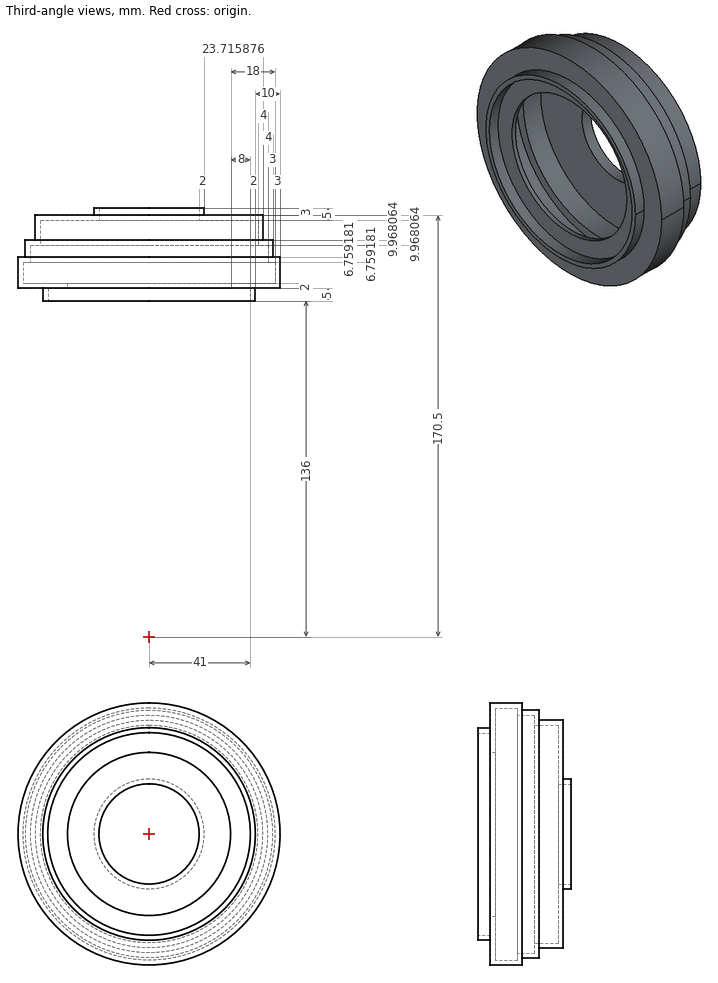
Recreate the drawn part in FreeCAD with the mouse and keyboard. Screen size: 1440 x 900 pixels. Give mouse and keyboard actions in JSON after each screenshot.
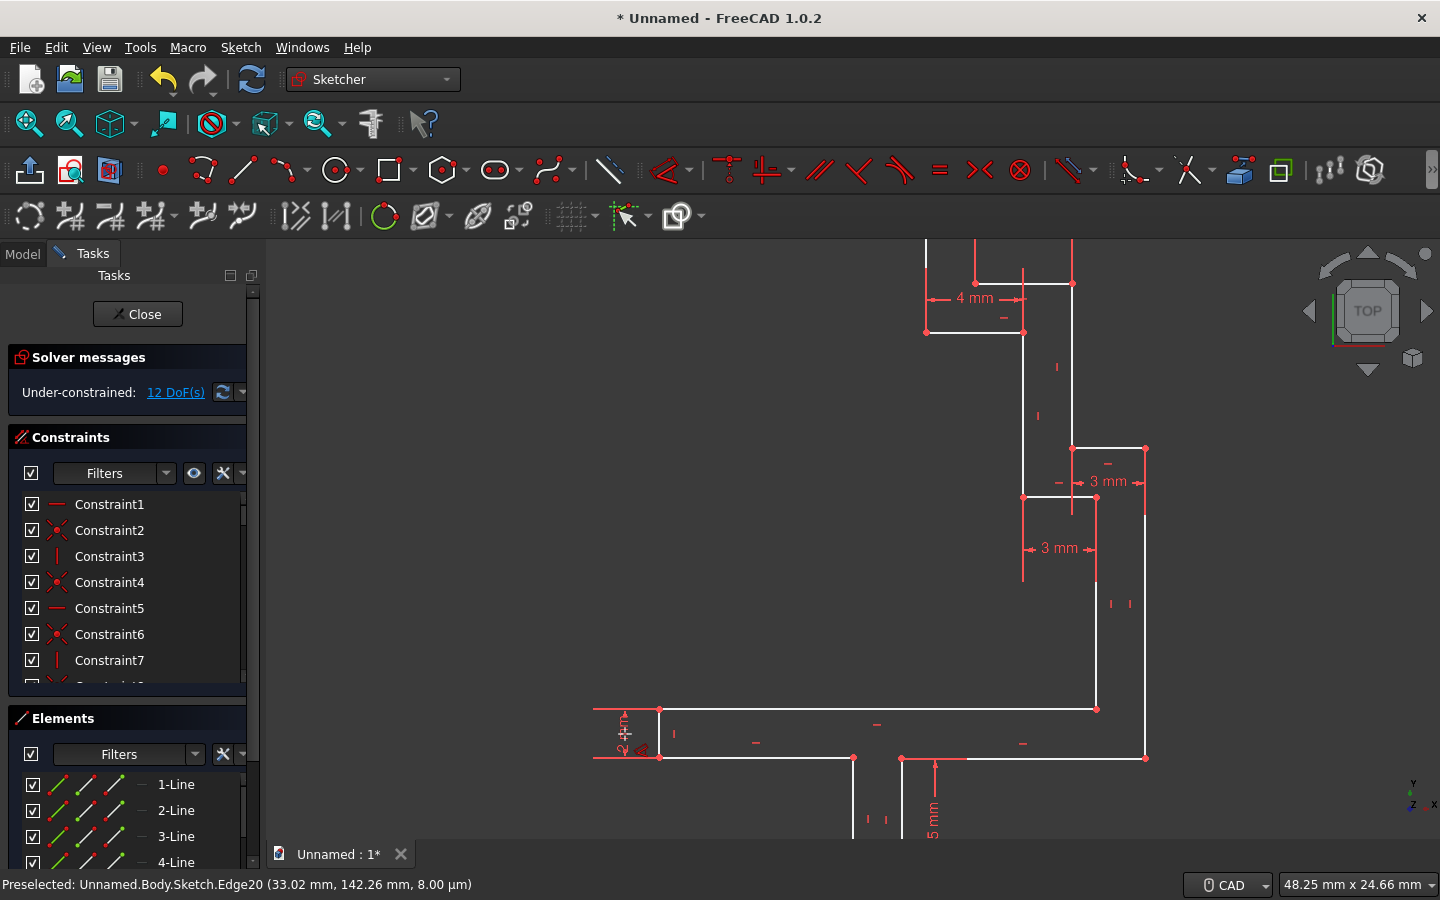
{"action": "left_click", "coordinate": [717, 758]}
{"action": "left_click", "coordinate": [756, 792]}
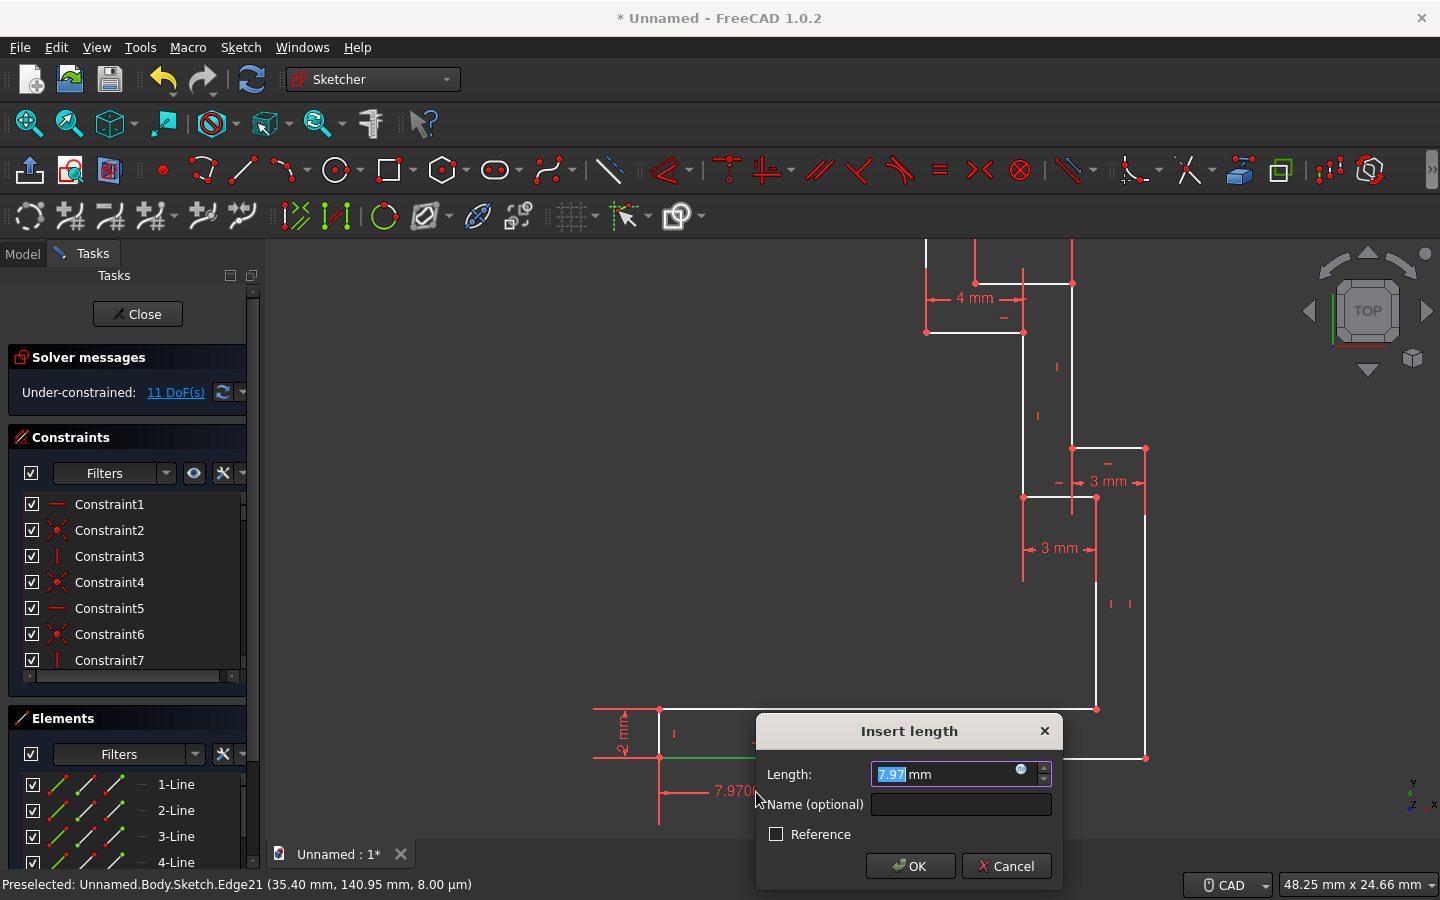
{"action": "type", "text": "8"}
{"action": "key", "text": "Return"}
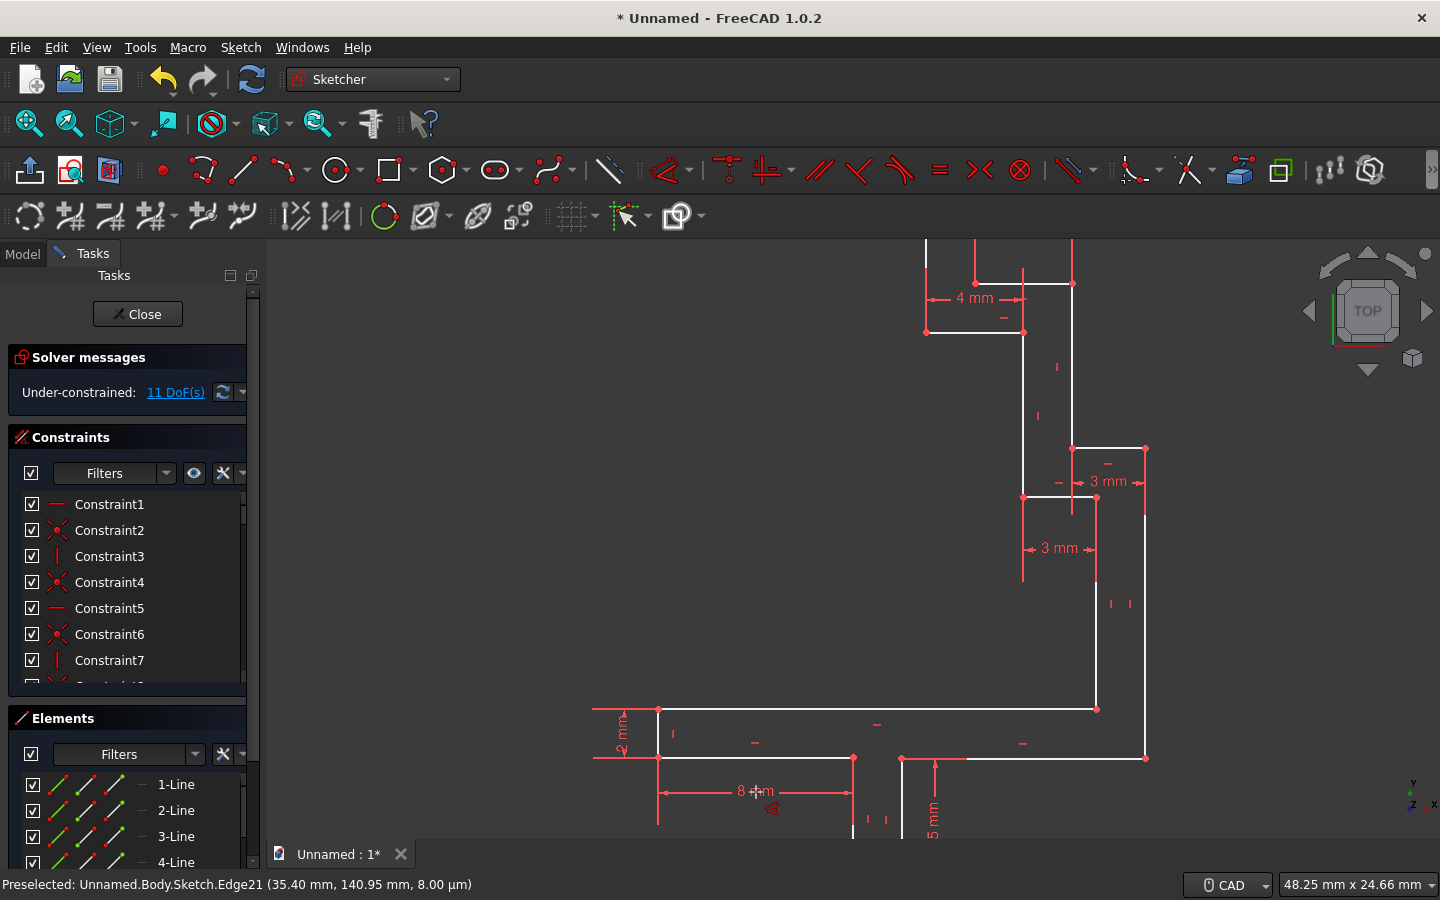
{"action": "left_click", "coordinate": [853, 794]}
{"action": "left_click", "coordinate": [887, 784]}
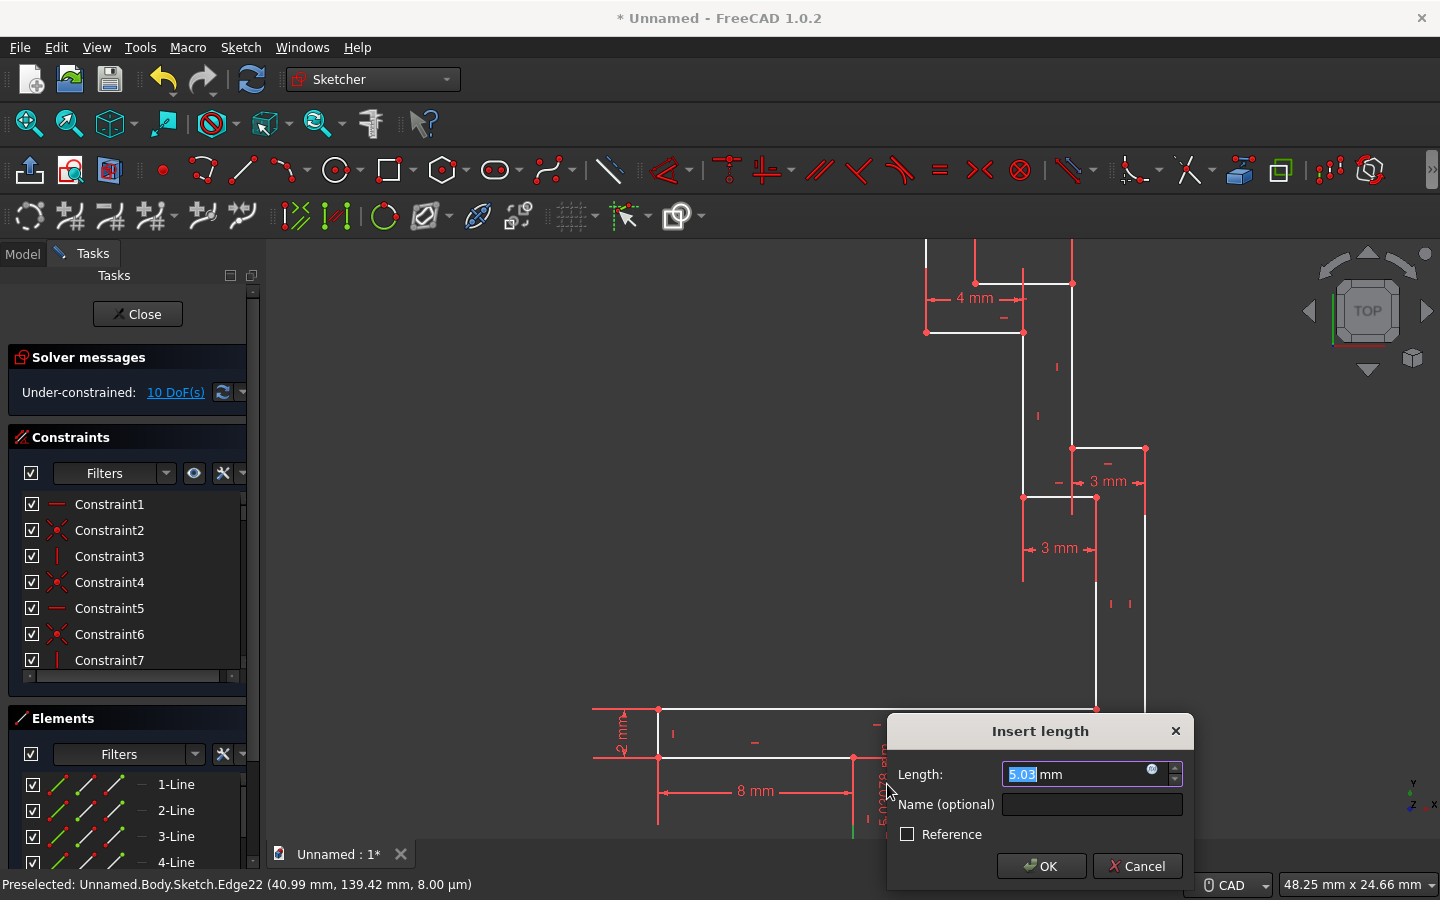
{"action": "type", "text": "5"}
{"action": "key", "text": "Return"}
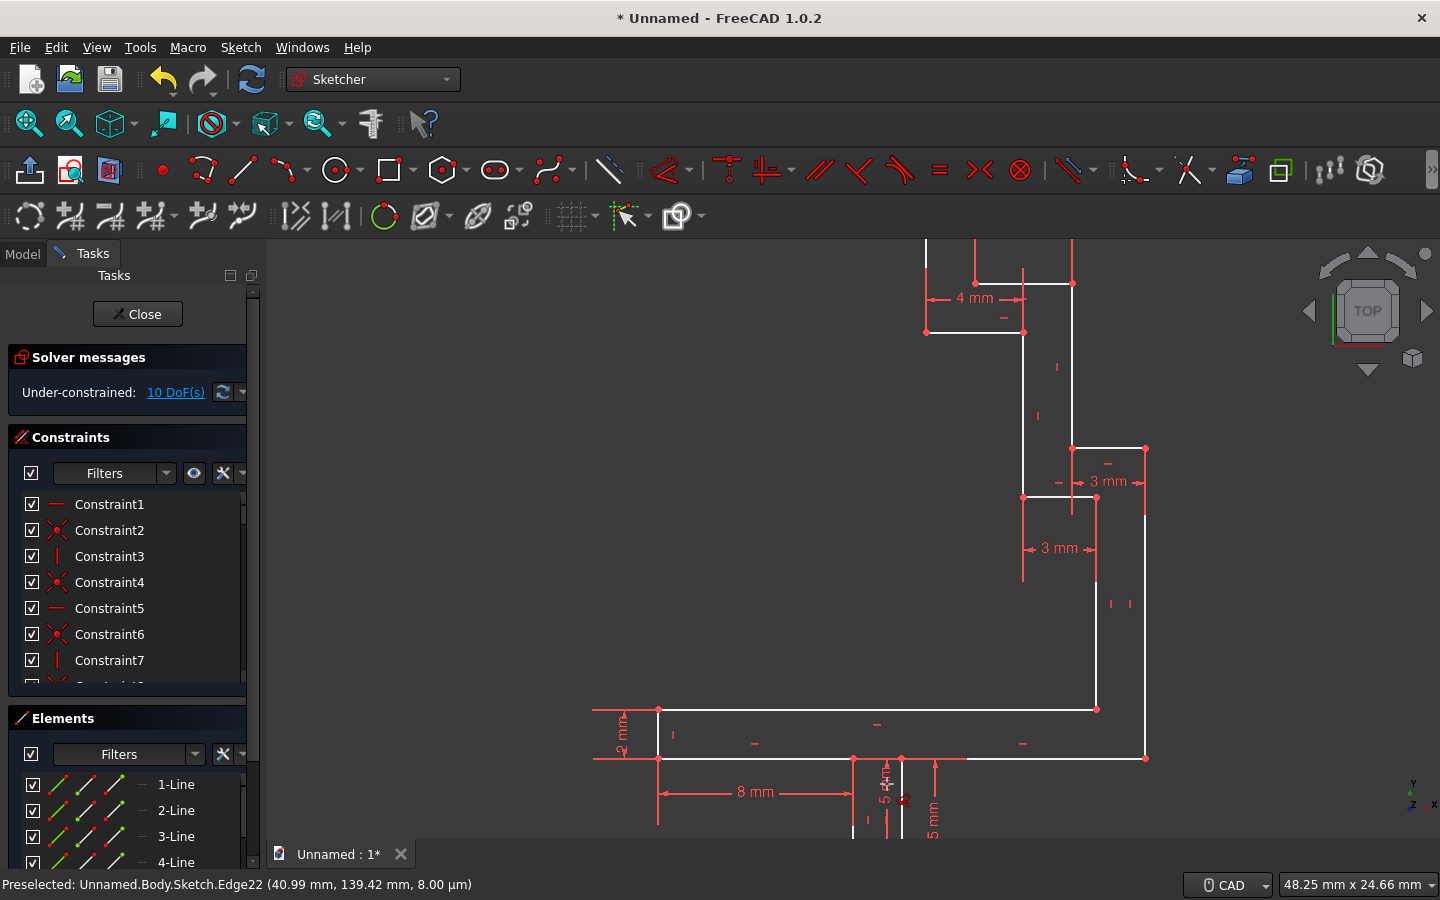
{"action": "left_click", "coordinate": [975, 759]}
{"action": "left_click", "coordinate": [1024, 793]}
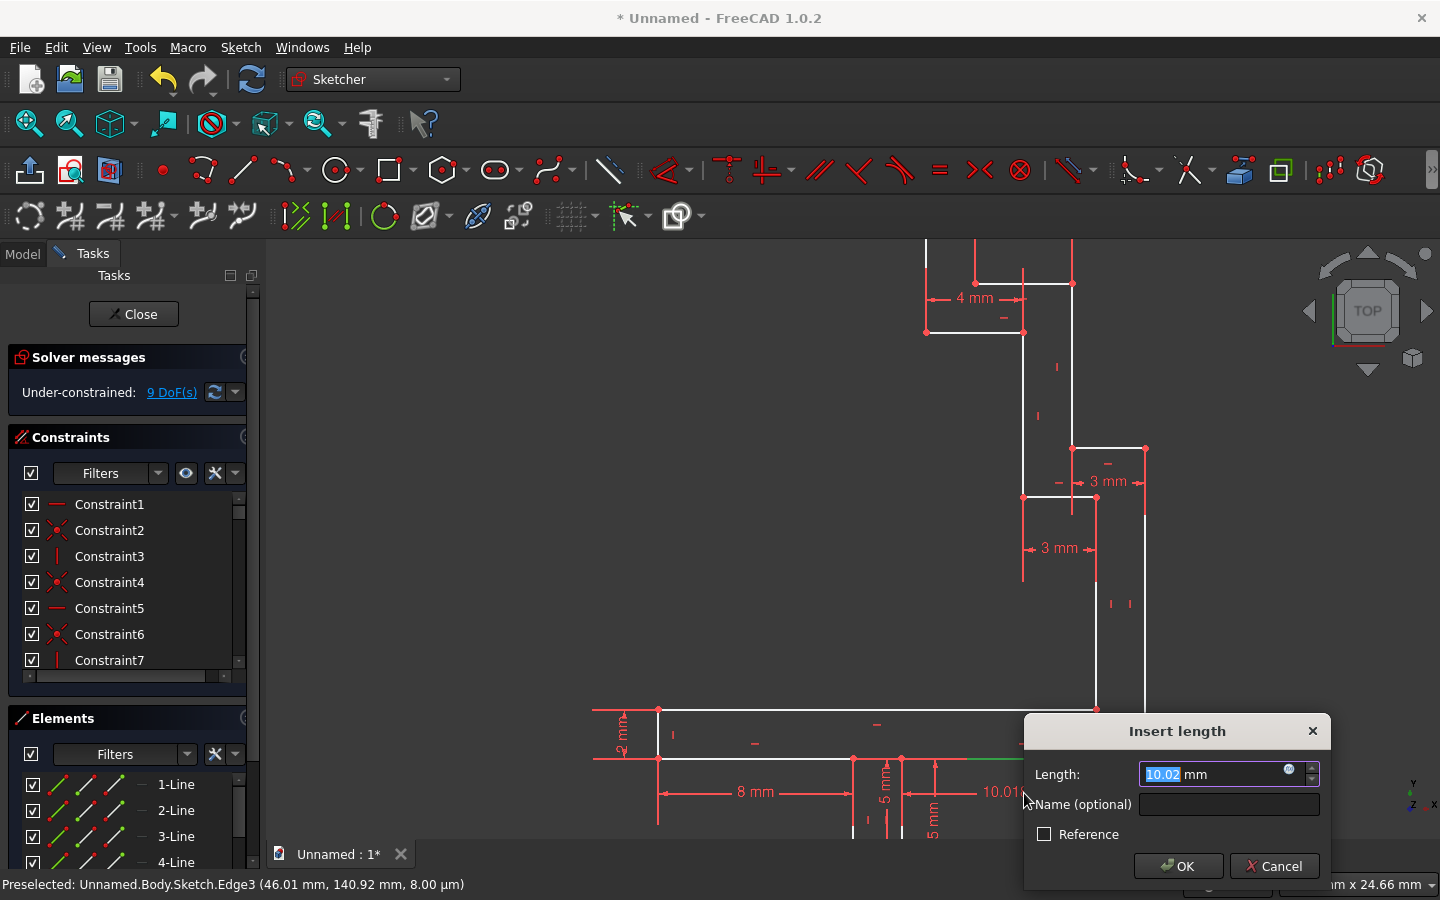
{"action": "type", "text": "10"}
{"action": "key", "text": "Return"}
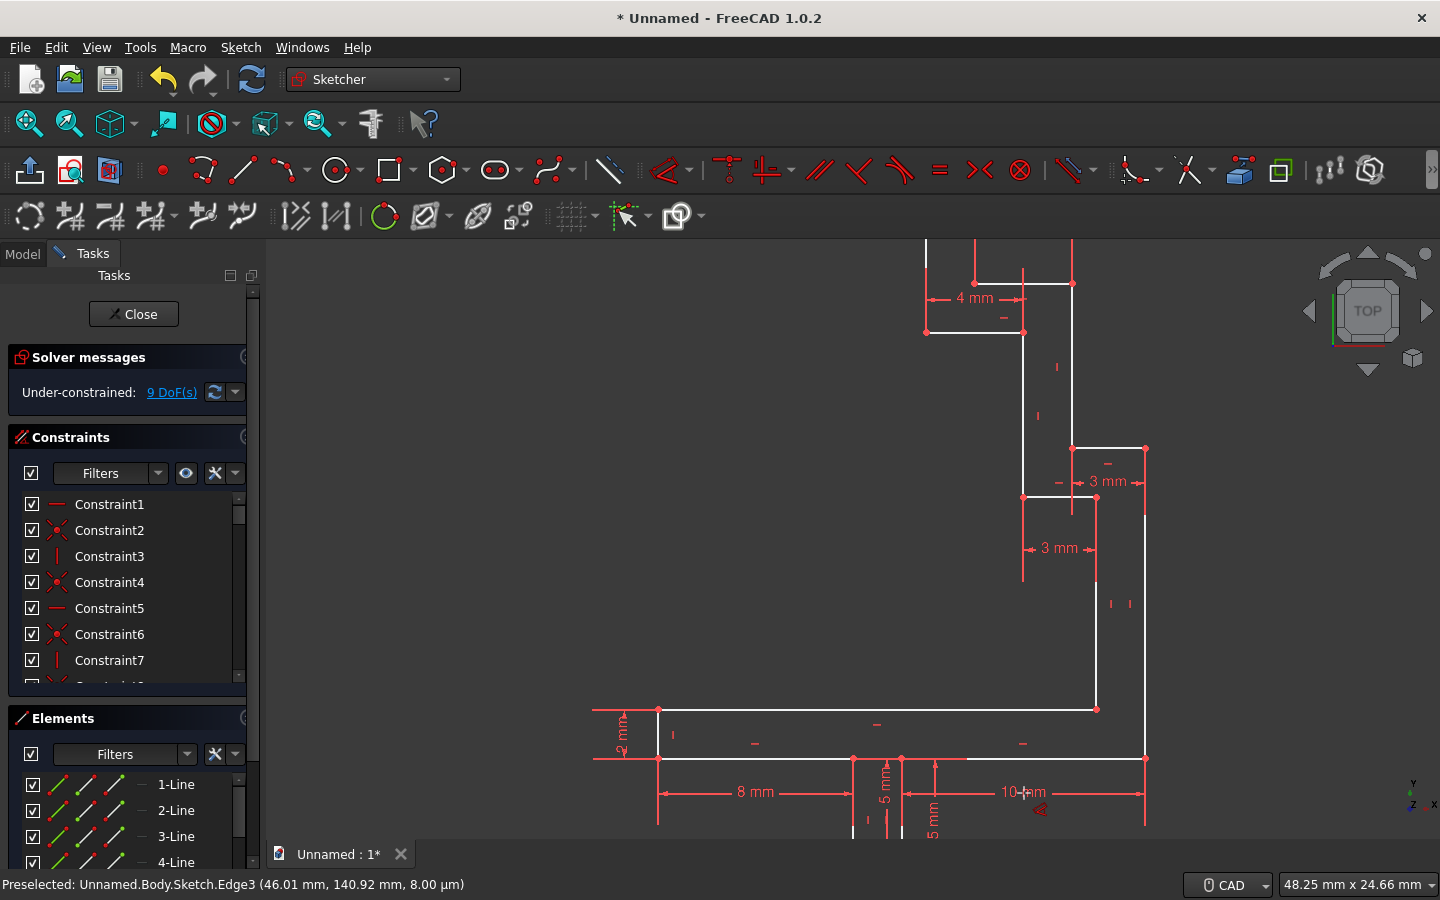
{"action": "left_click", "coordinate": [965, 710]}
{"action": "left_click", "coordinate": [877, 744]}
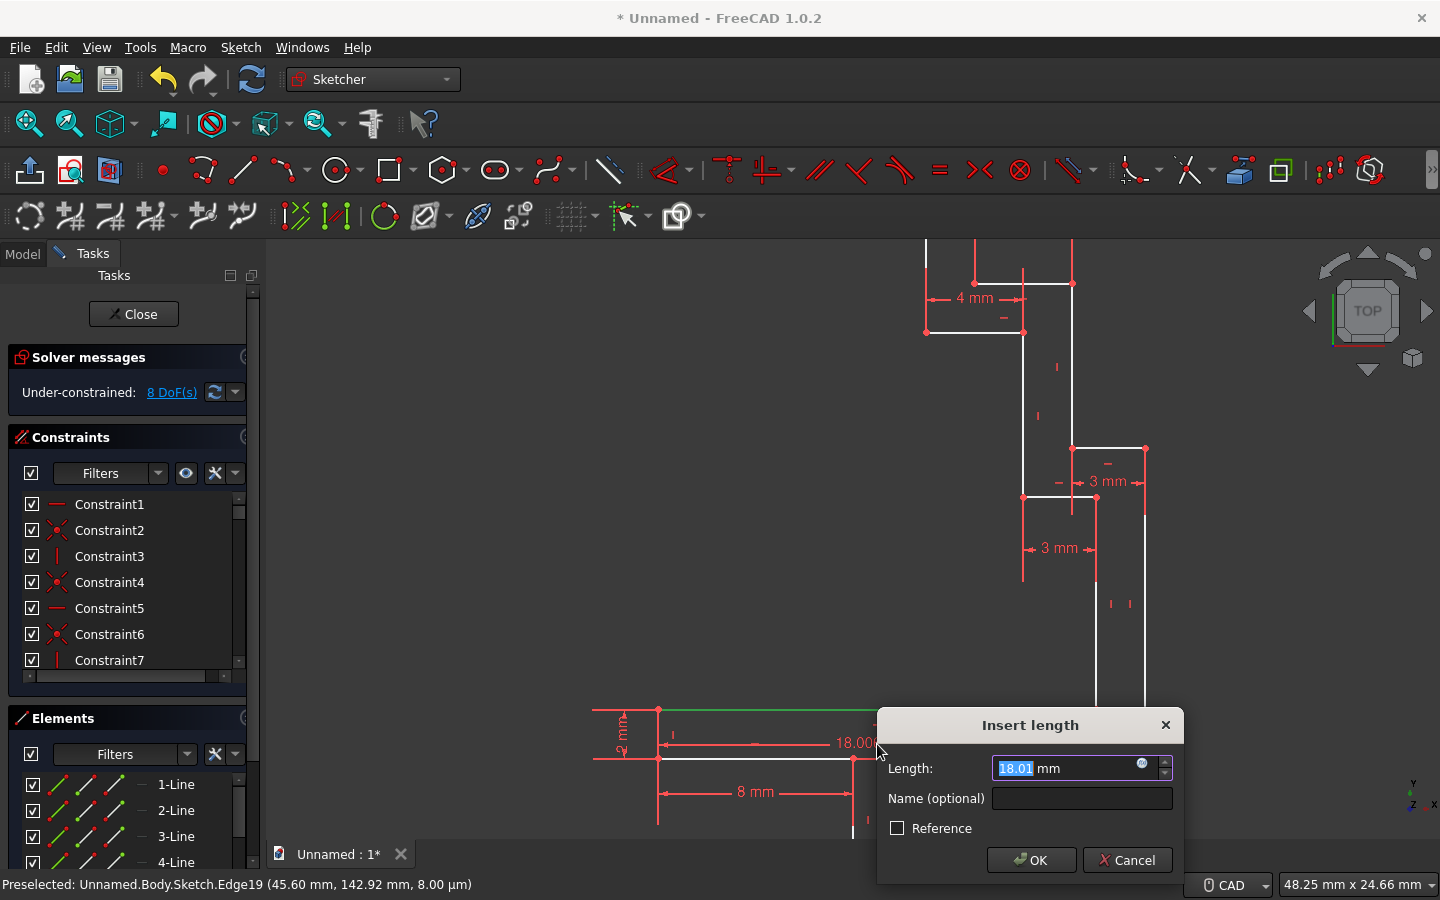
{"action": "type", "text": "18"}
{"action": "key", "text": "Return"}